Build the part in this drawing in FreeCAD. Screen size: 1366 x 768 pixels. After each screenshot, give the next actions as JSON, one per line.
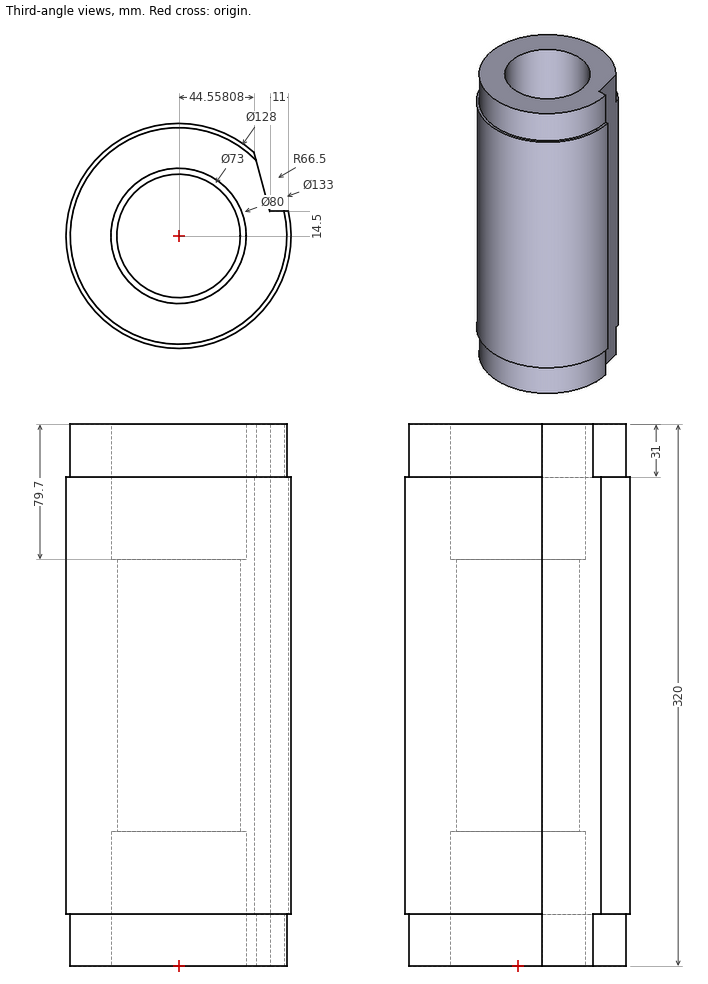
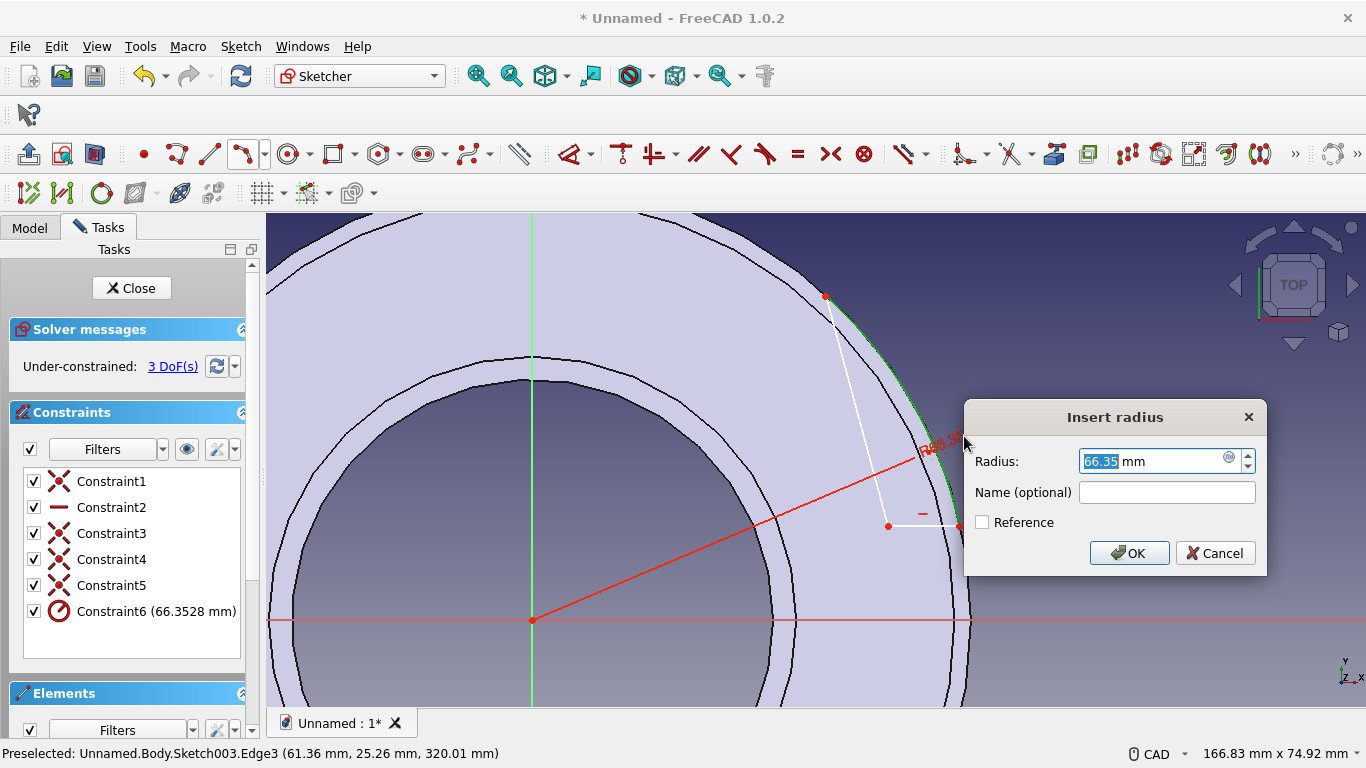
{"action": "type", "text": "66.5"}
{"action": "key", "text": "Return"}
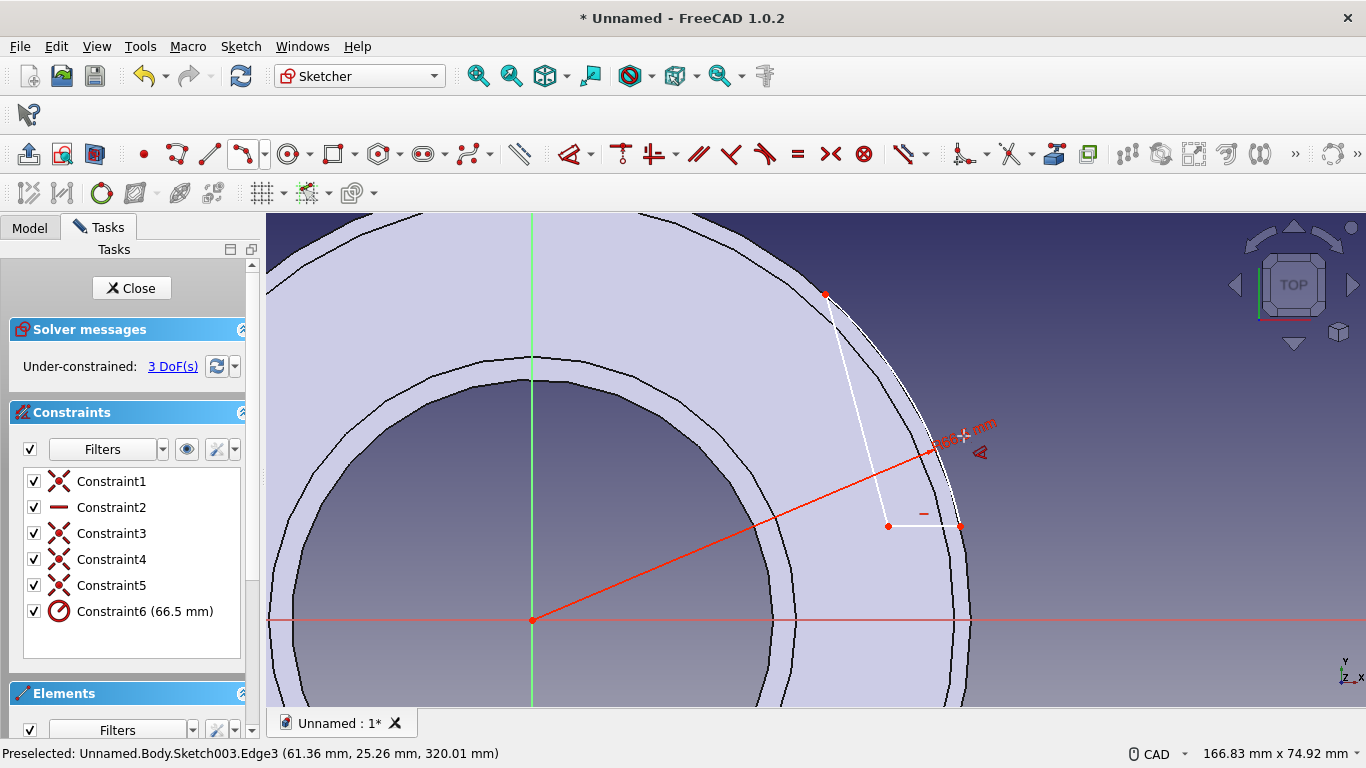
{"action": "left_click", "coordinate": [910, 526]}
{"action": "left_click", "coordinate": [924, 560]}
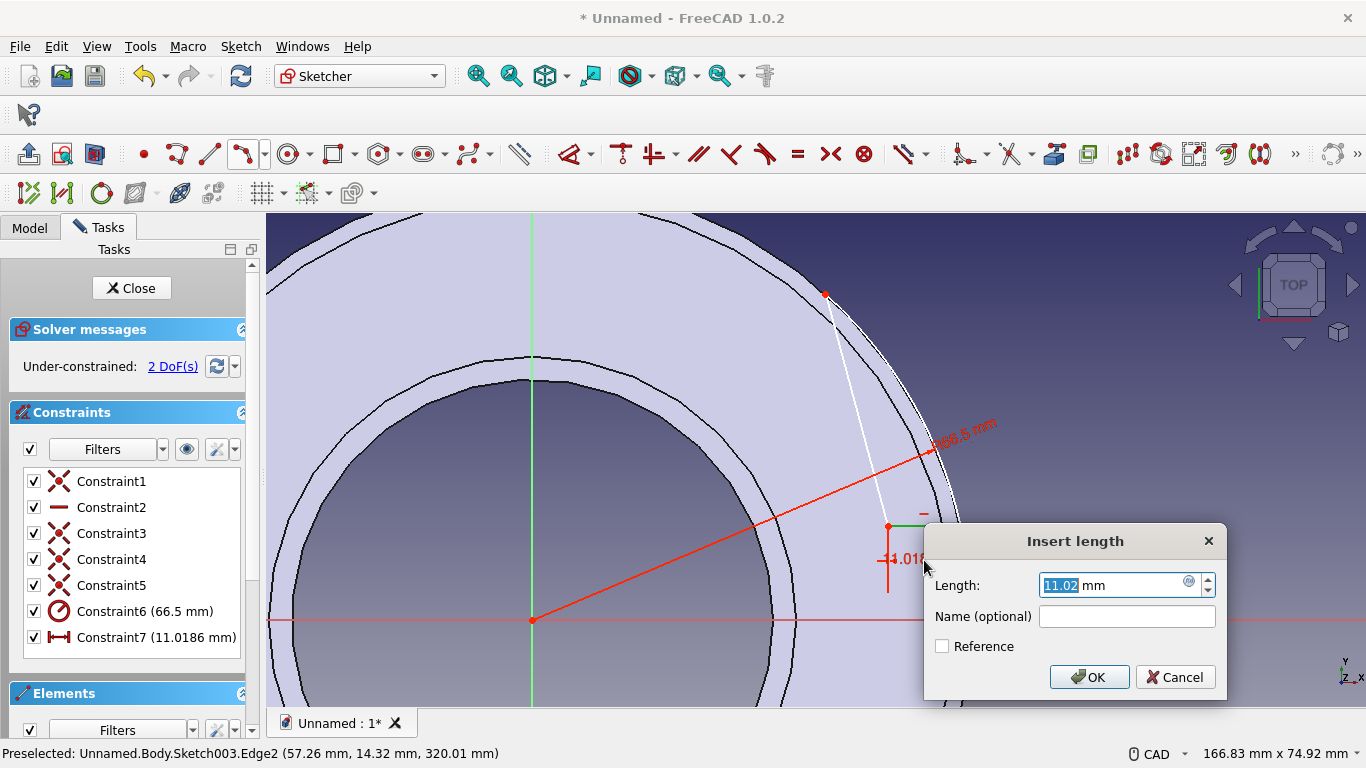
{"action": "type", "text": "11"}
{"action": "key", "text": "Return"}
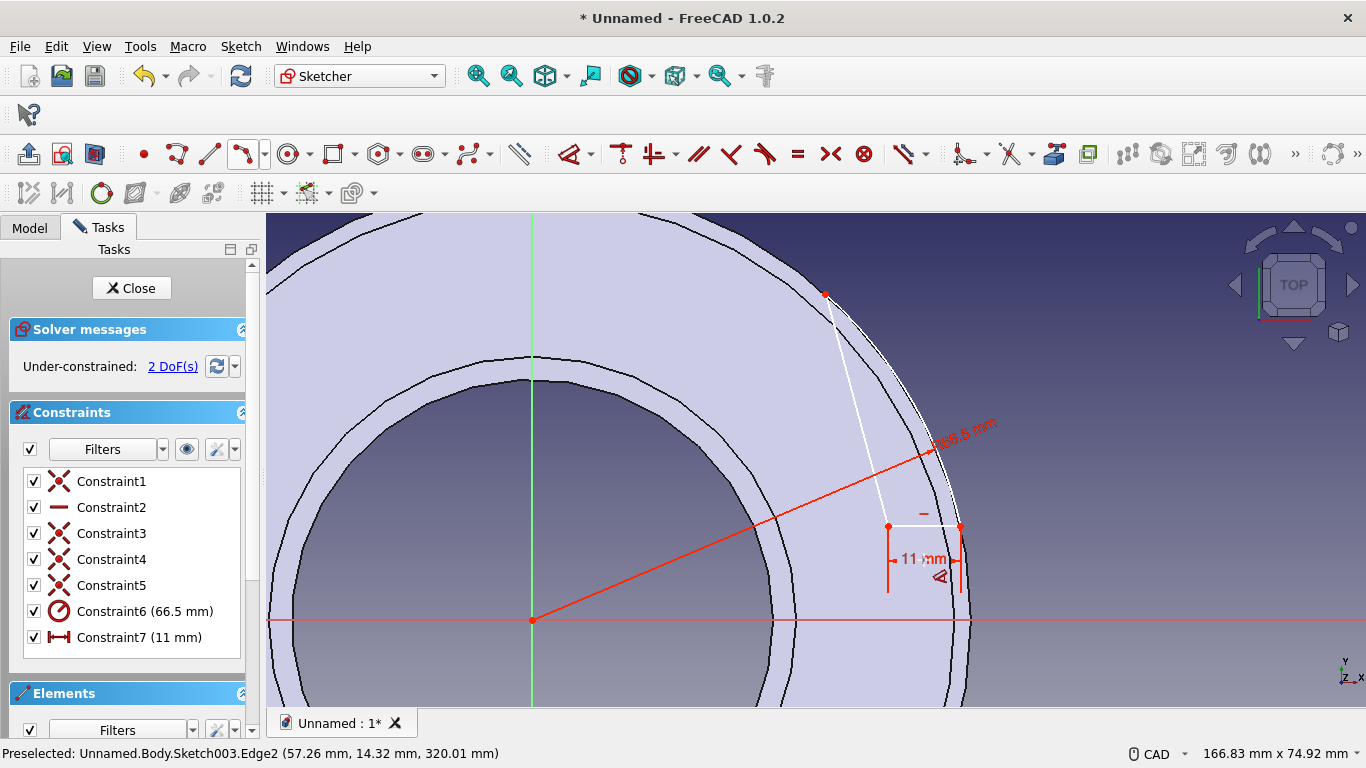
{"action": "left_click", "coordinate": [888, 526]}
{"action": "left_click", "coordinate": [498, 573]}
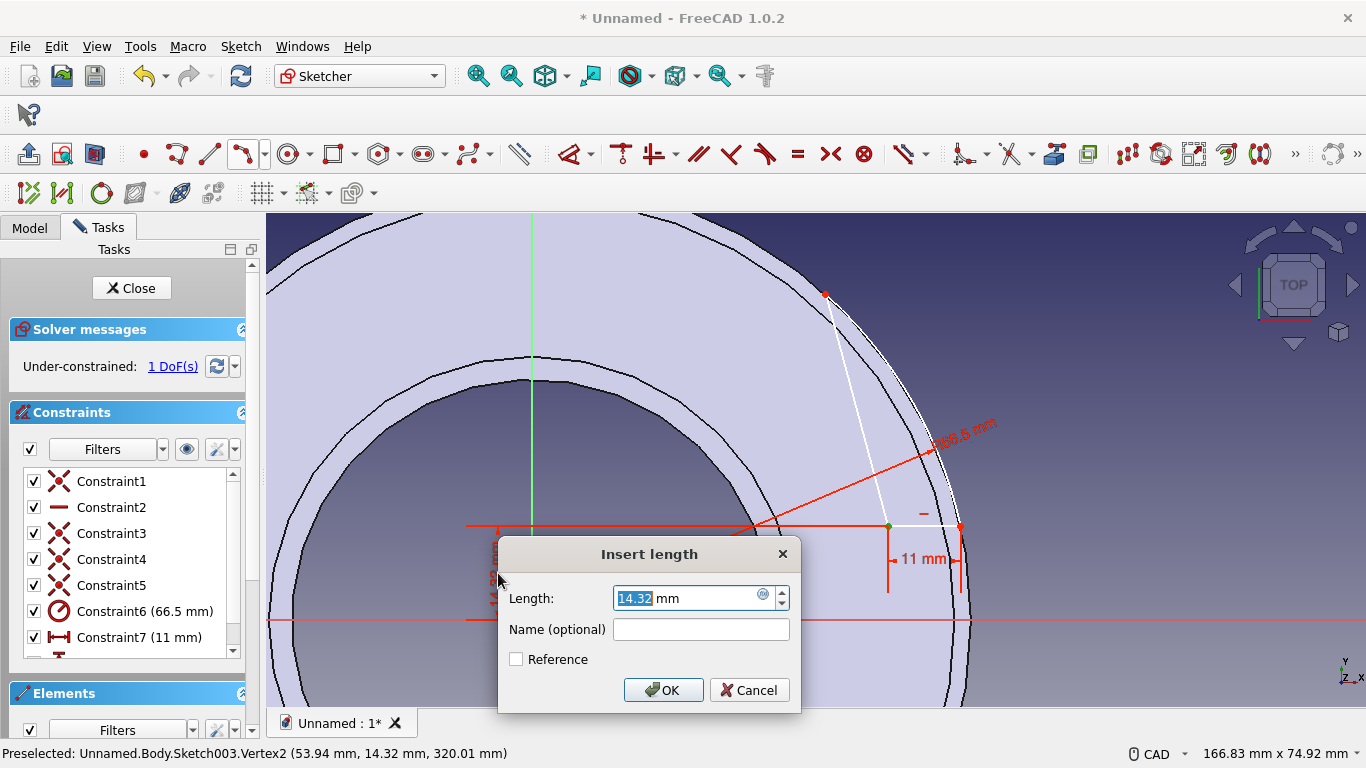
{"action": "type", "text": "14.5"}
{"action": "key", "text": "Return"}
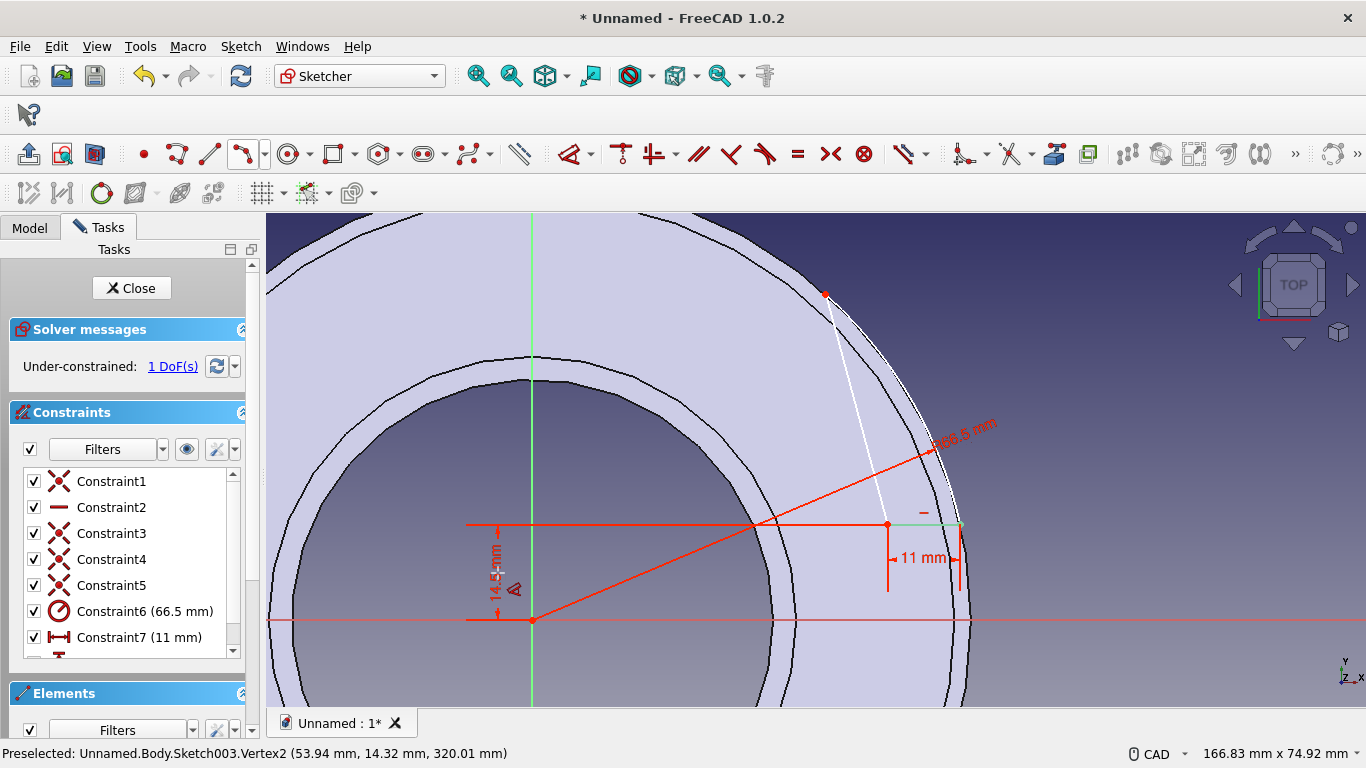
{"action": "left_click", "coordinate": [826, 295]}
{"action": "left_click", "coordinate": [679, 261]}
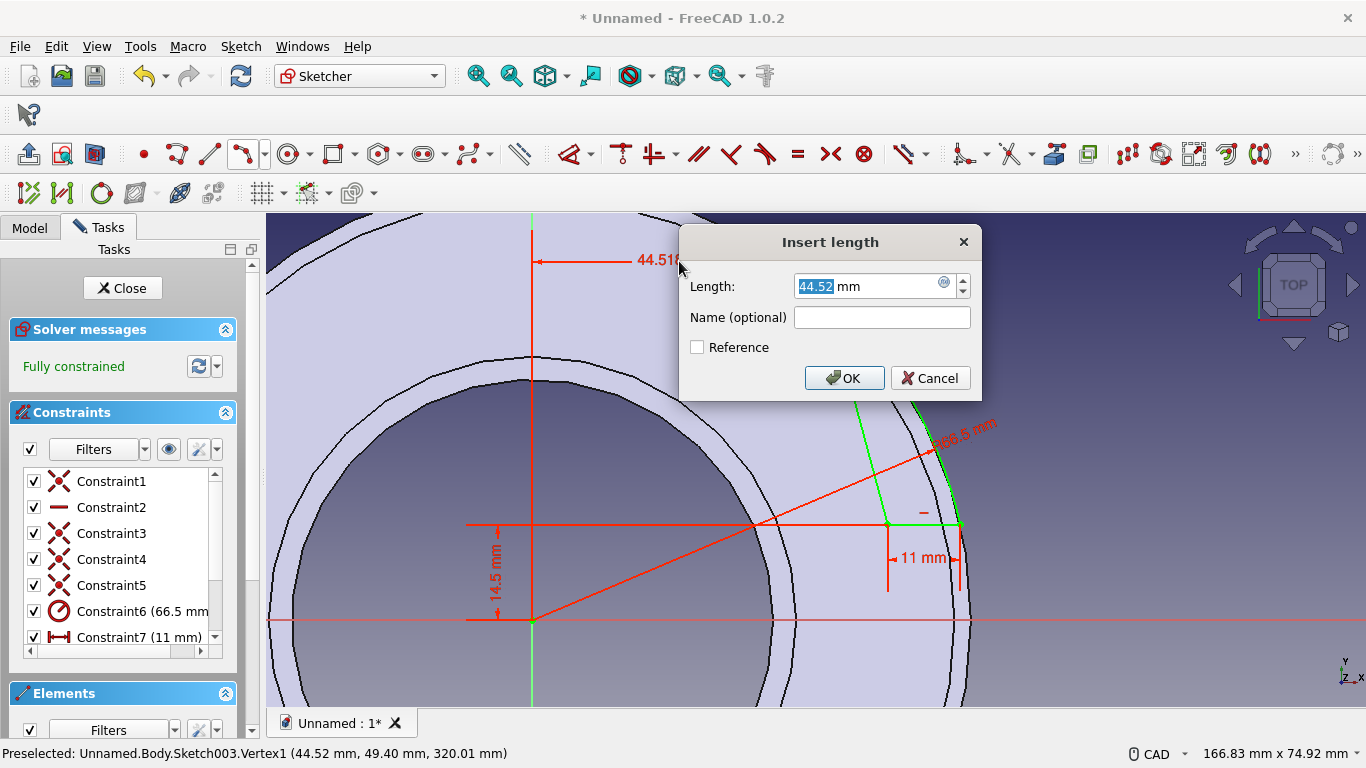
{"action": "type", "text": "44.55808"}
{"action": "key", "text": "Return"}
{"action": "key", "text": "Escape"}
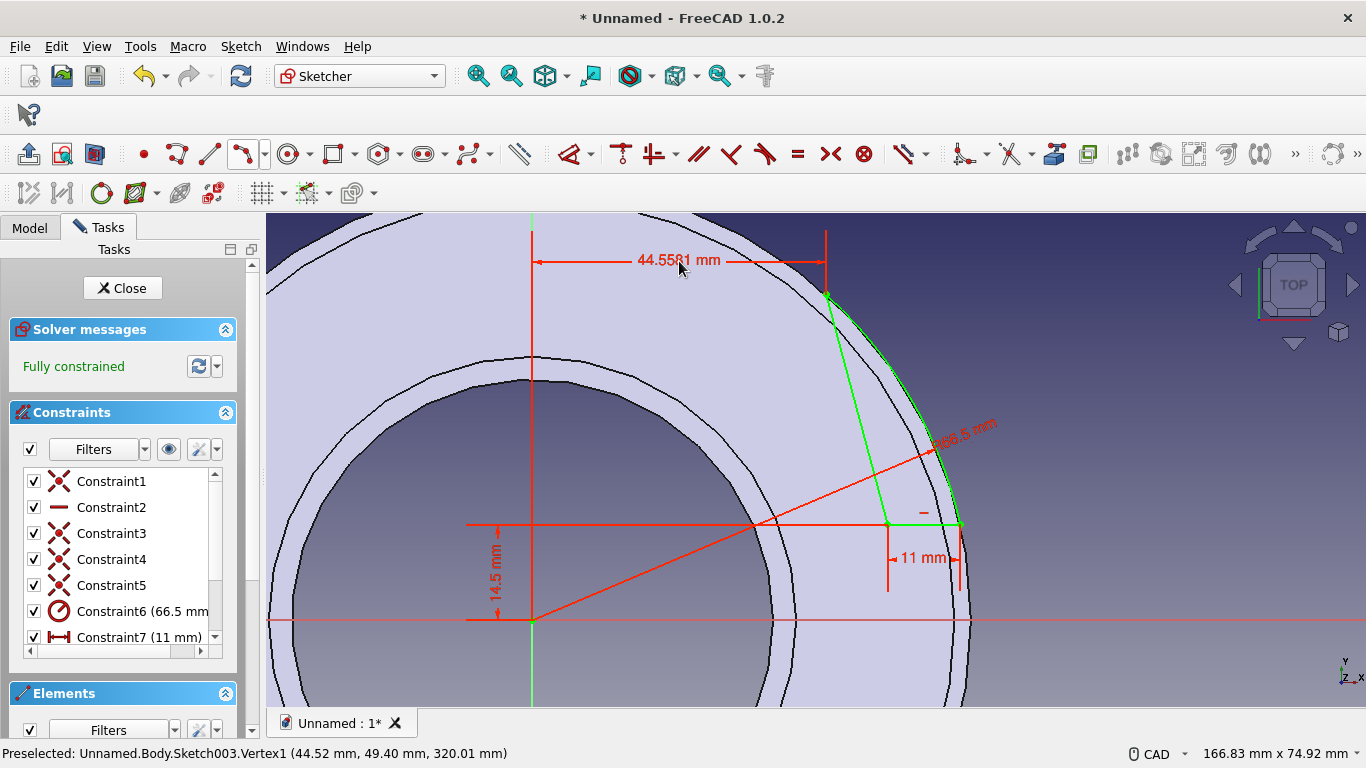
{"action": "left_click", "coordinate": [123, 288]}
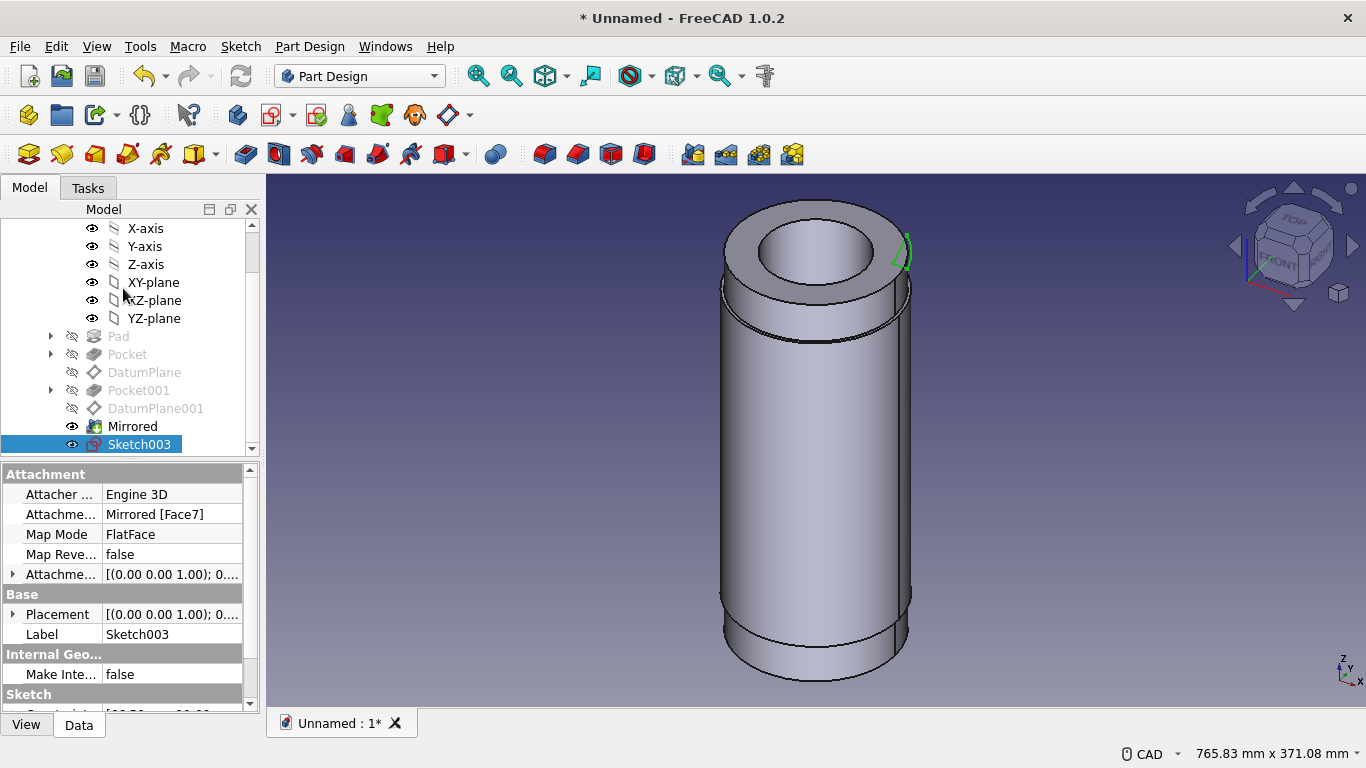
{"action": "left_click", "coordinate": [246, 154]}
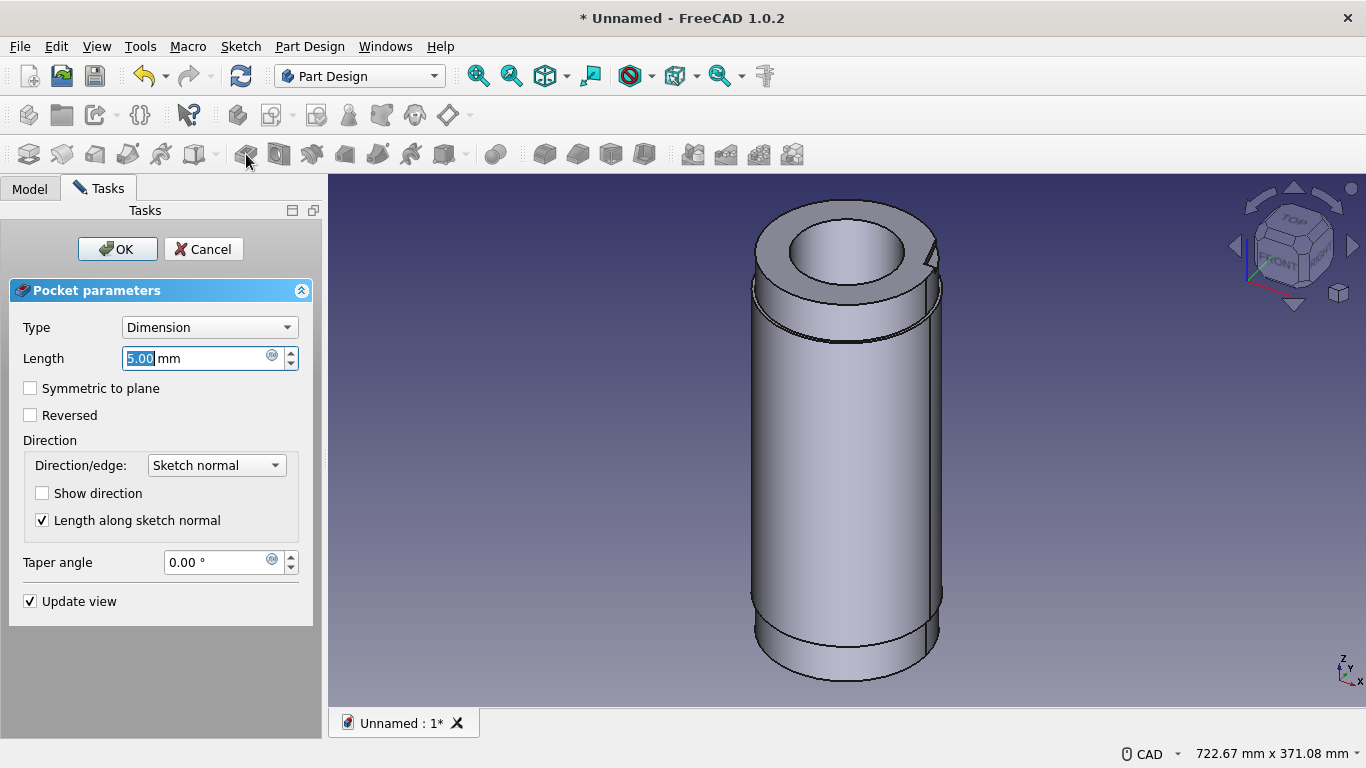
{"action": "left_click", "coordinate": [210, 328]}